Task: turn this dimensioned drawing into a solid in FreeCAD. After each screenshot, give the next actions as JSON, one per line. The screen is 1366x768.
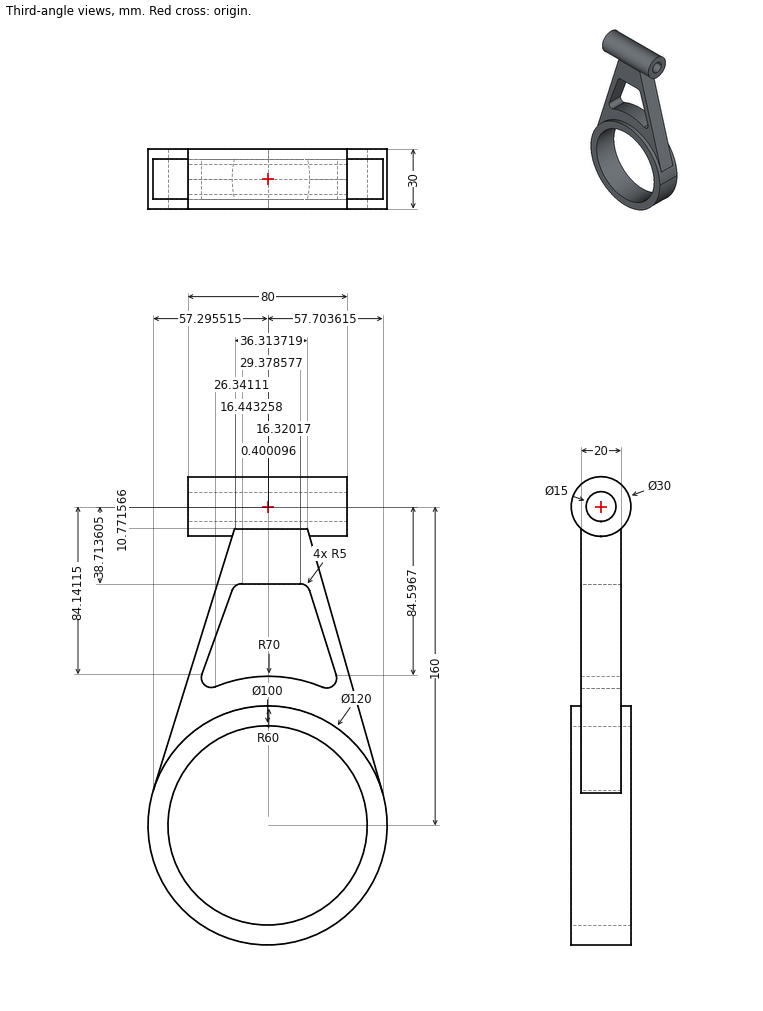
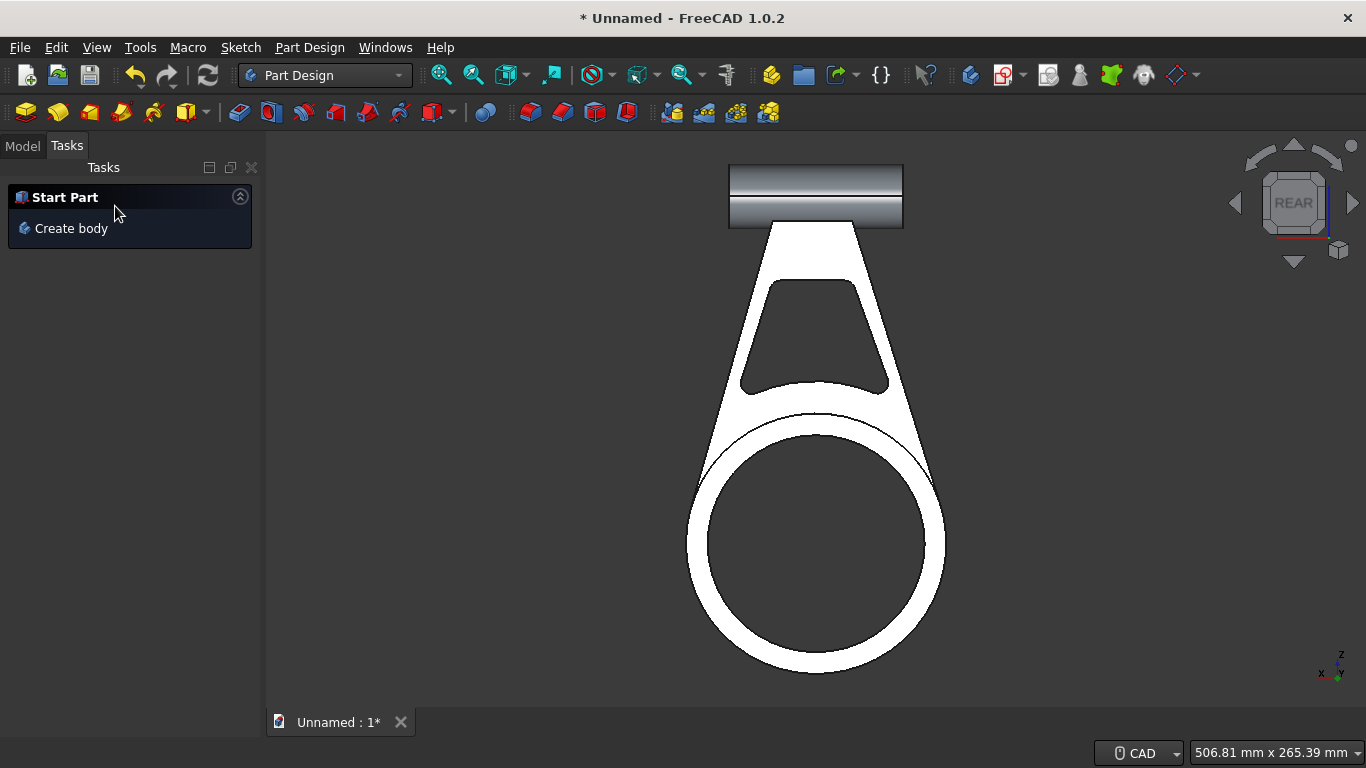
{"action": "key", "text": "0"}